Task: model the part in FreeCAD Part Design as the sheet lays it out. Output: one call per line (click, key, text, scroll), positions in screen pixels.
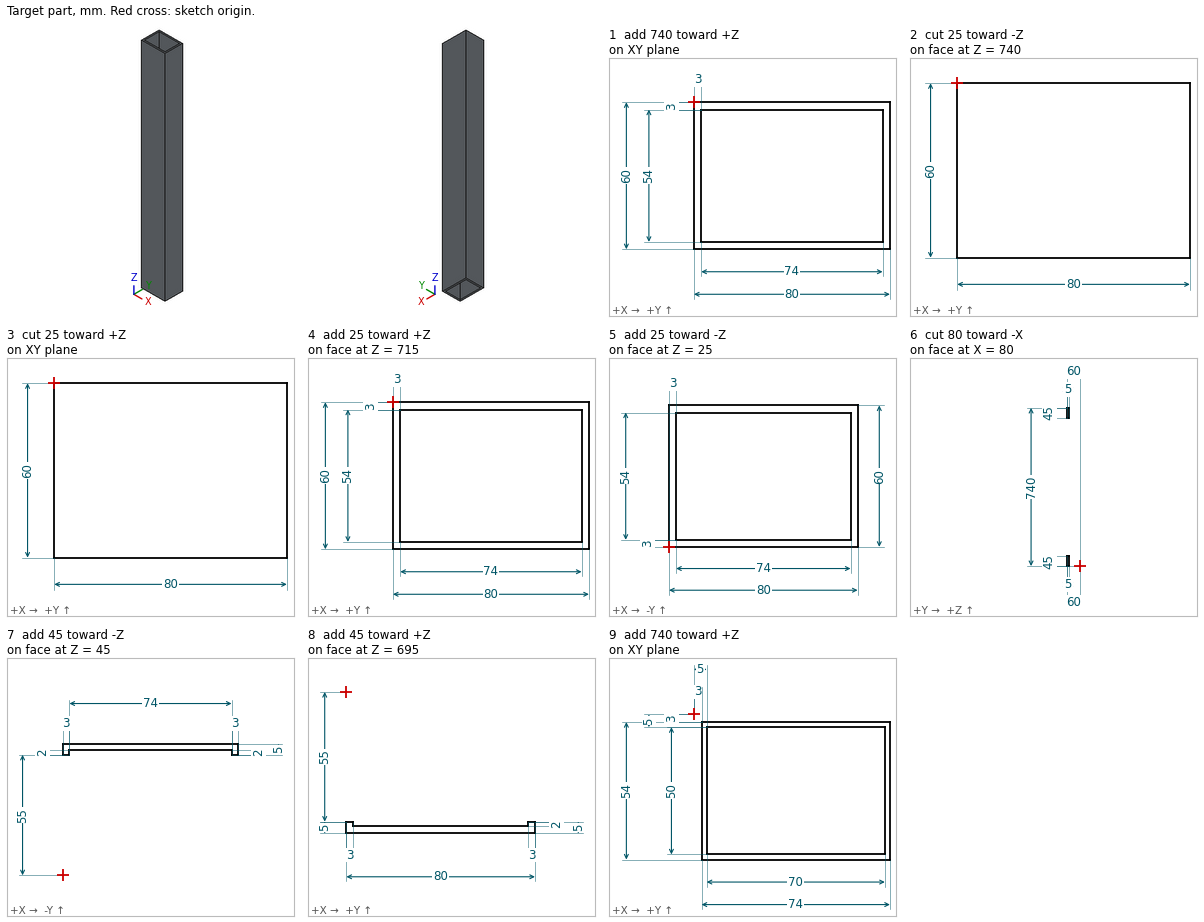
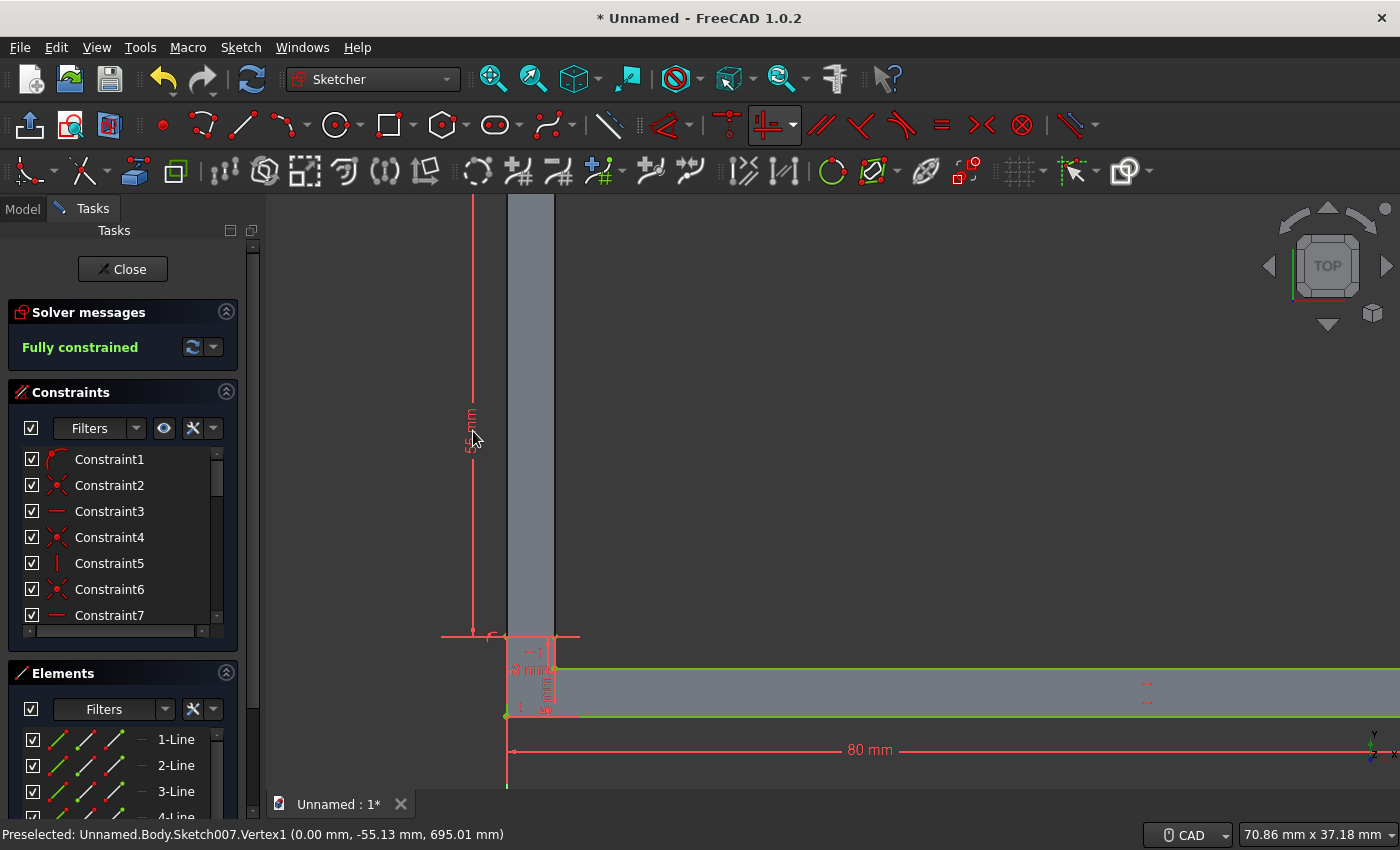
click(123, 269)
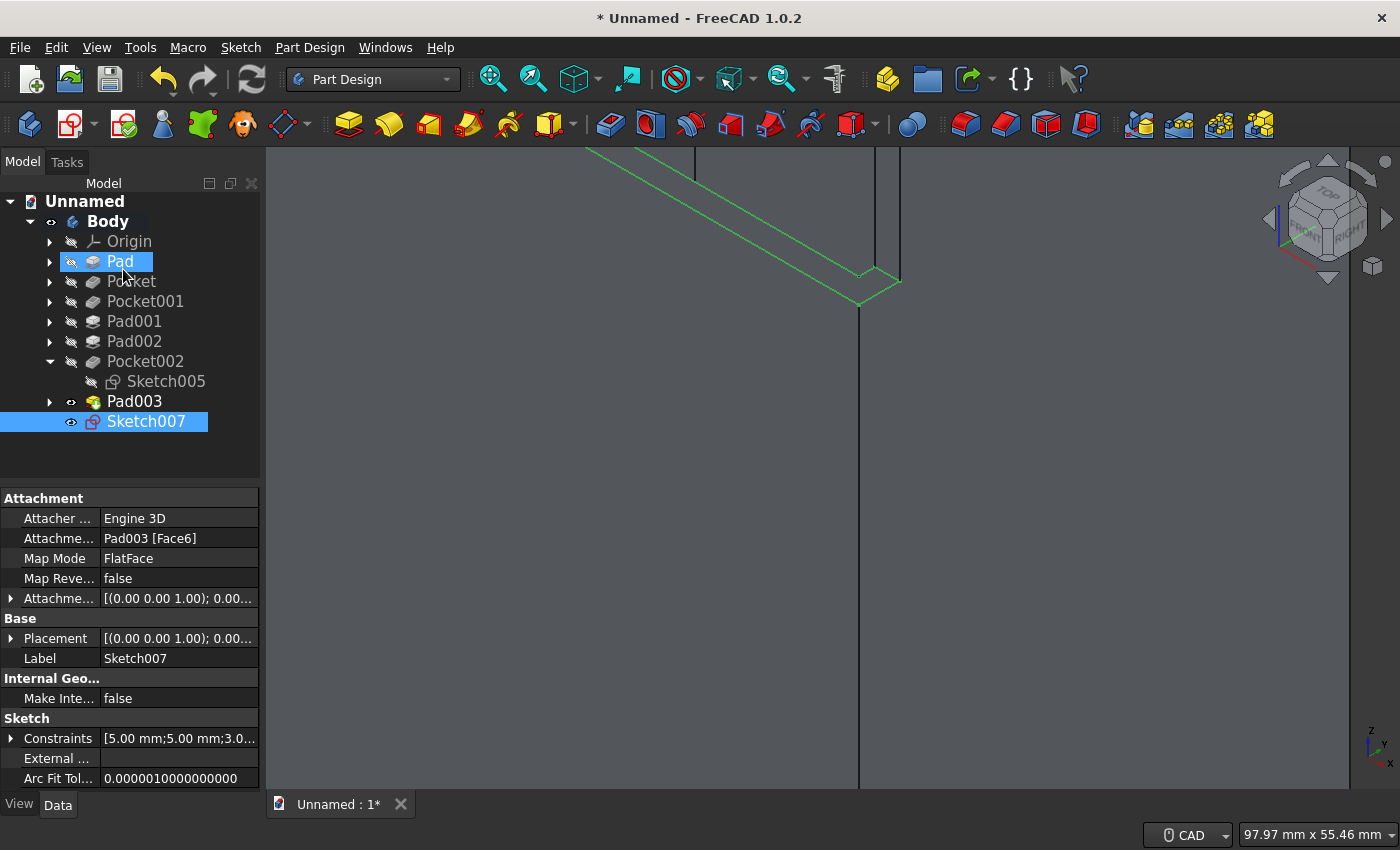
click(350, 124)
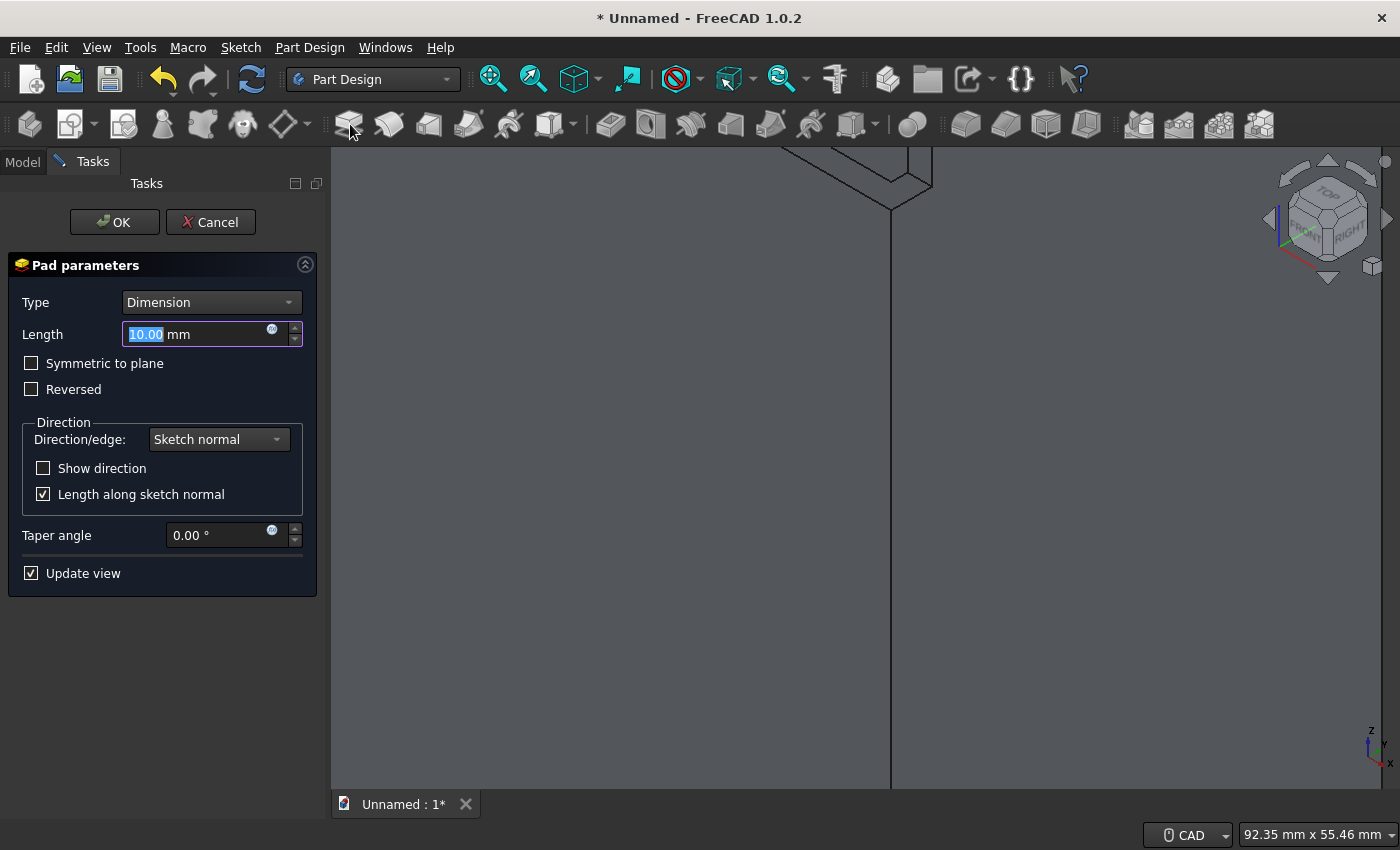
text(45)
key(Tab)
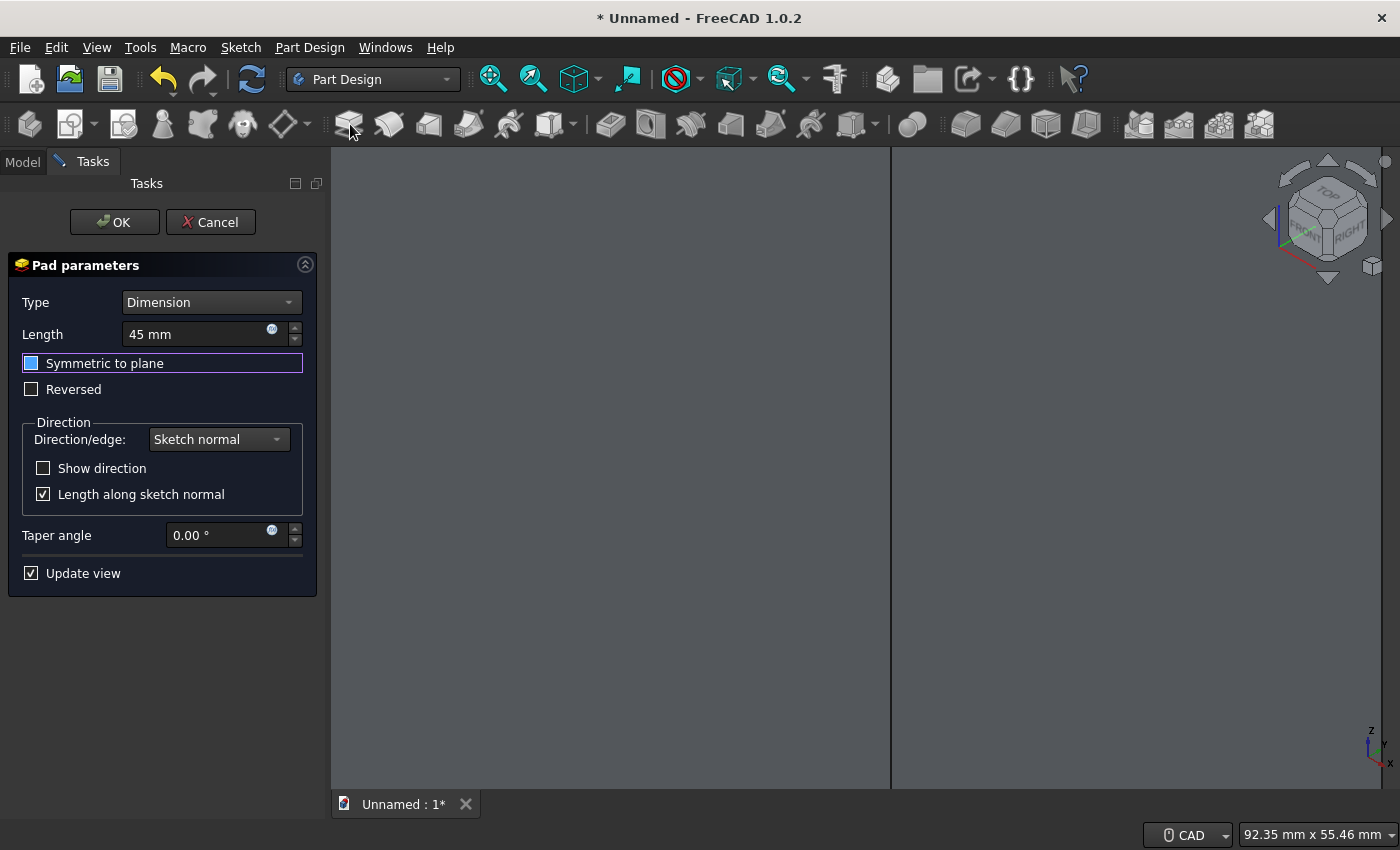
click(115, 222)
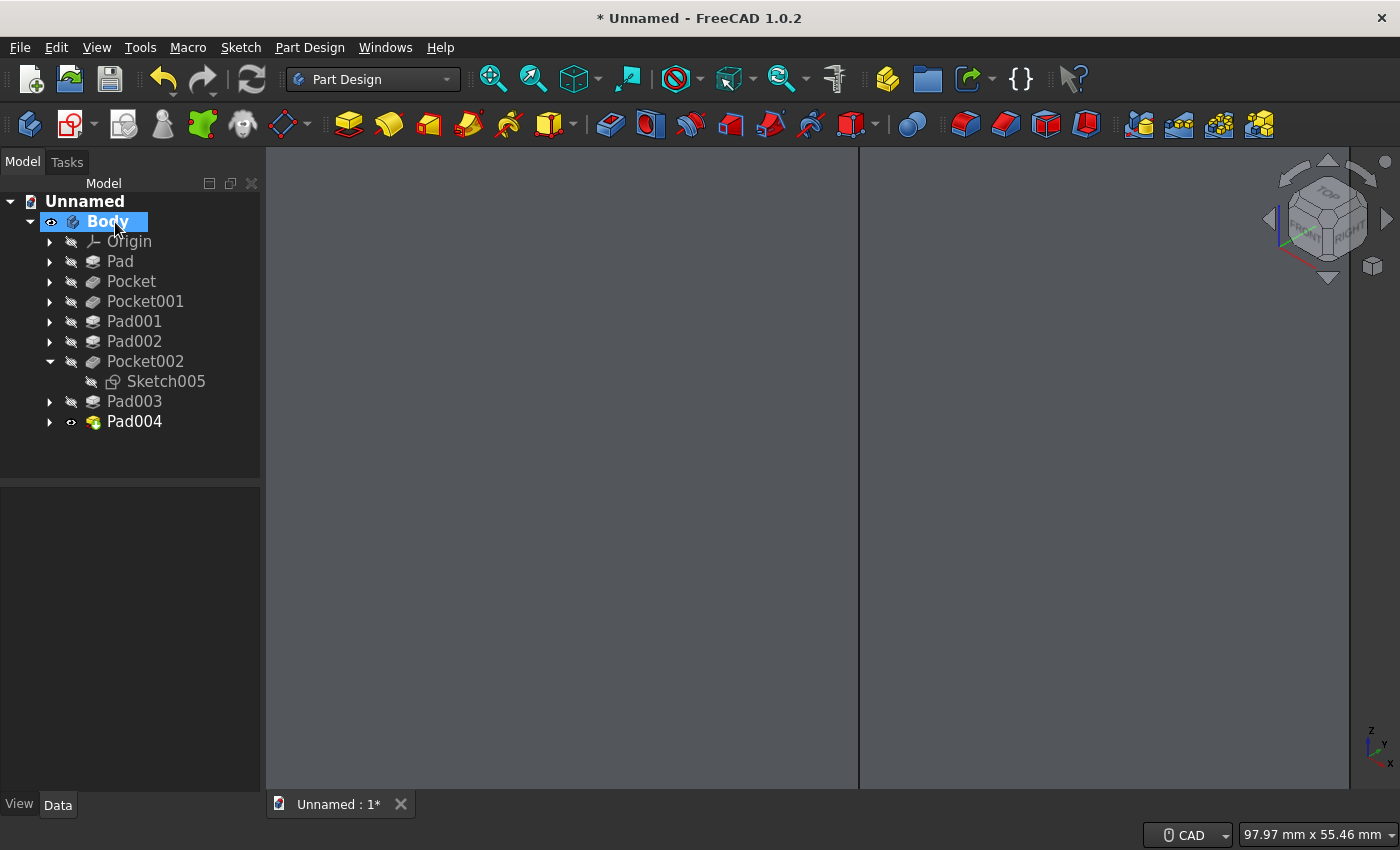
key(v)
key(f)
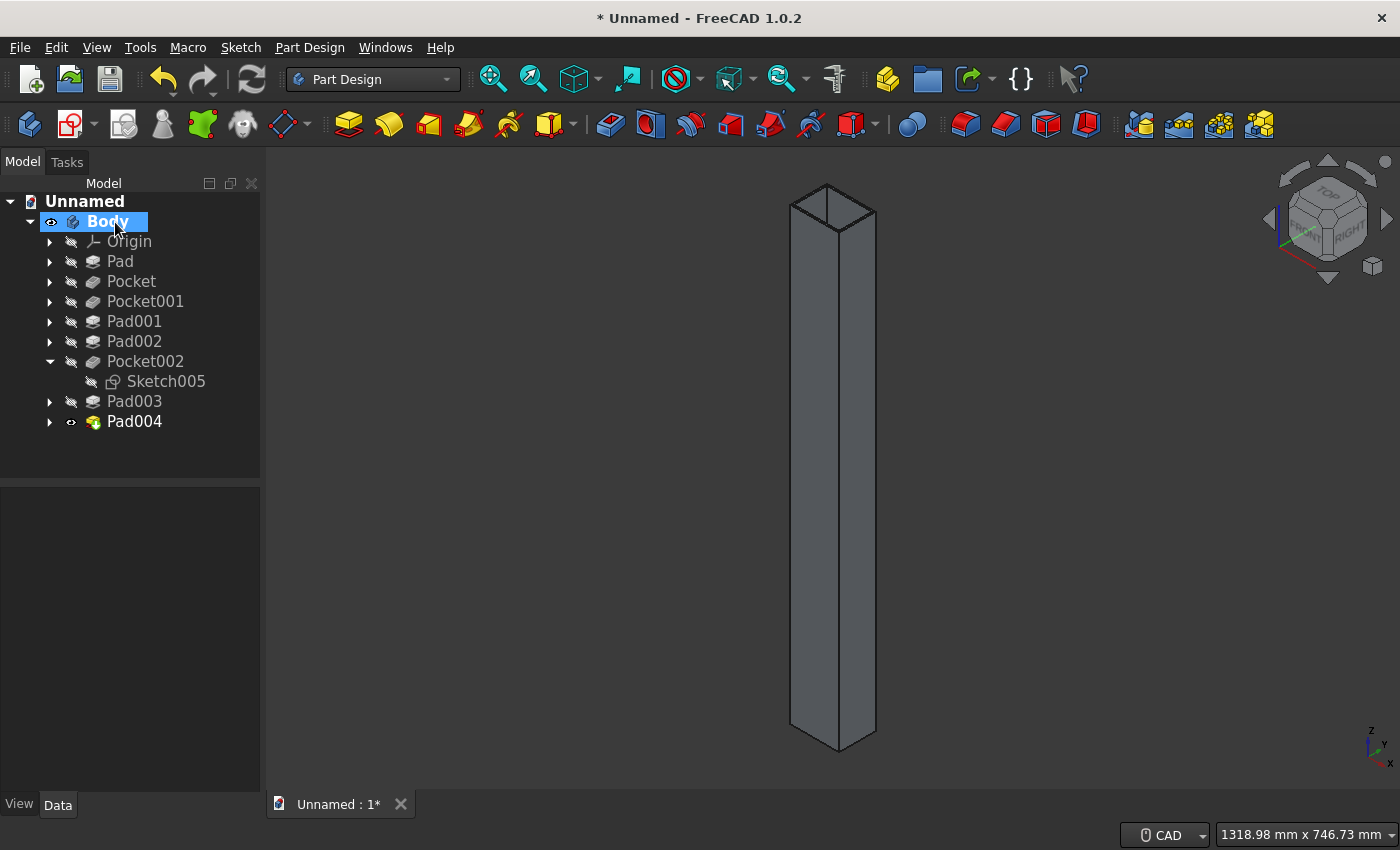
click(70, 124)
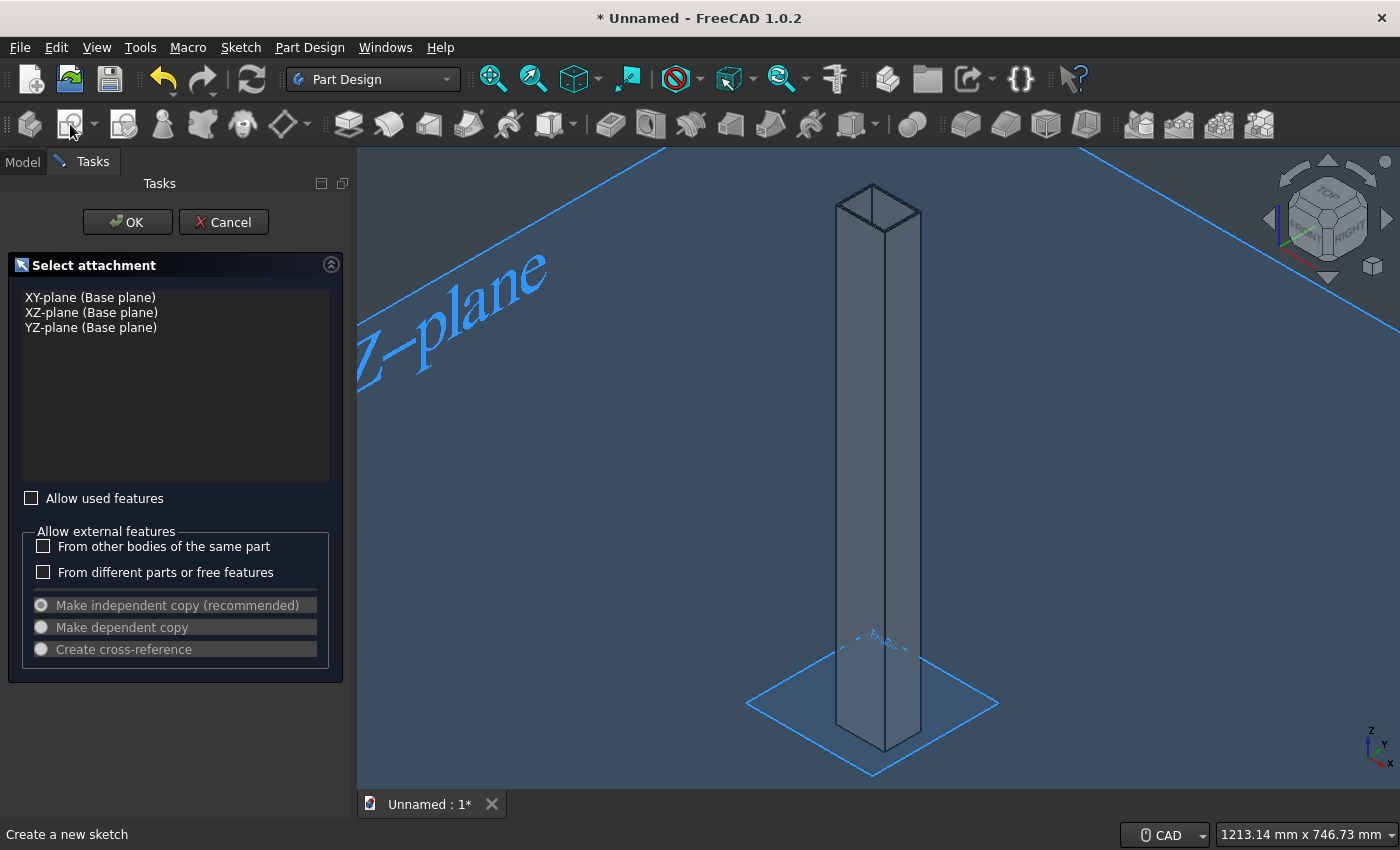
click(82, 298)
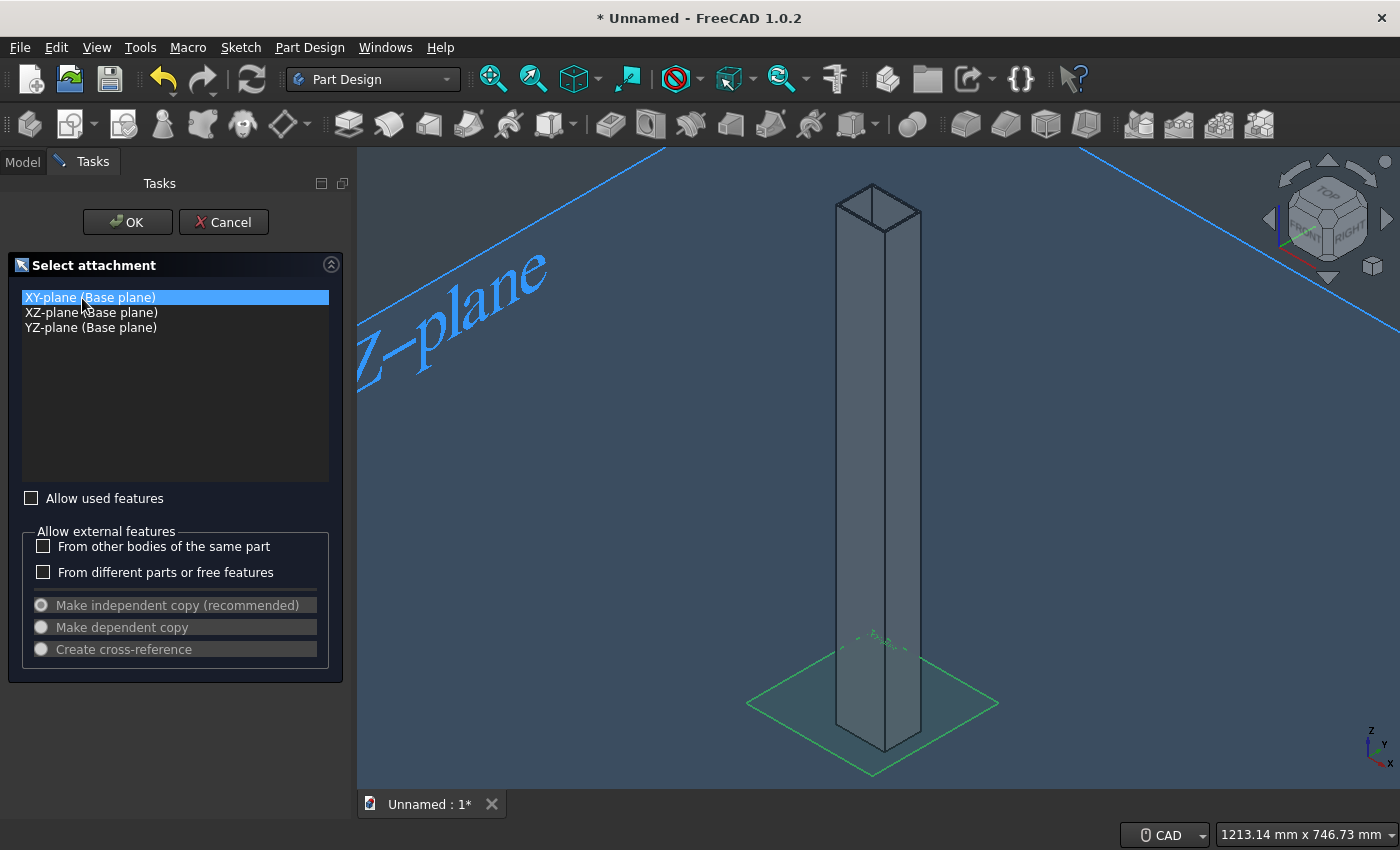
click(128, 222)